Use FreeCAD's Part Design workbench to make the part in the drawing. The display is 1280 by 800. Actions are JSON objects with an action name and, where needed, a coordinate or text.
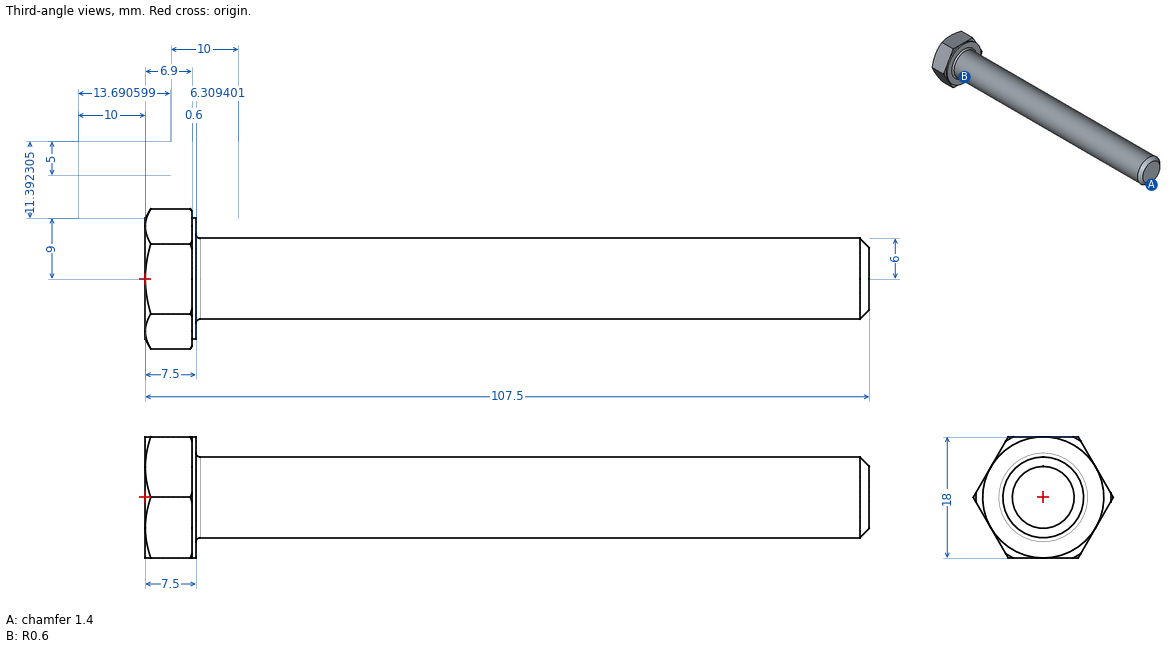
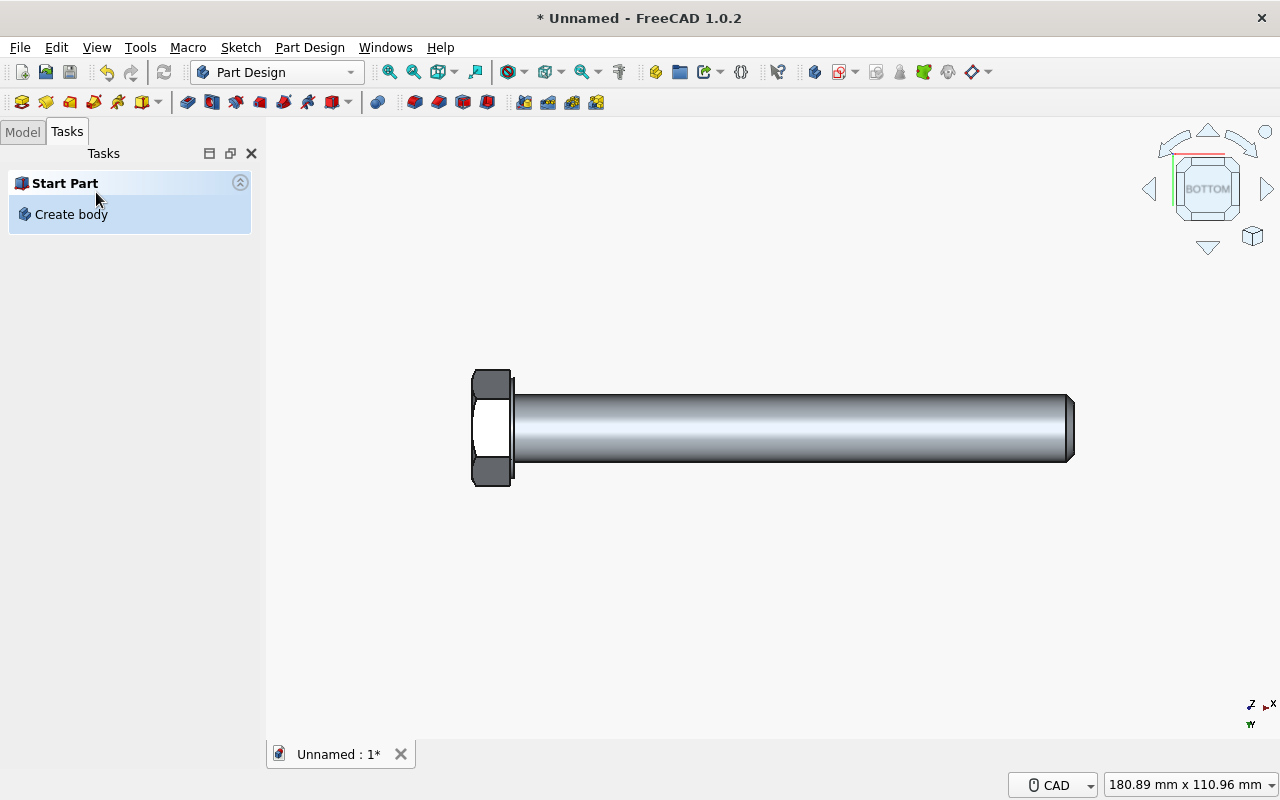
{"action": "key", "text": "4"}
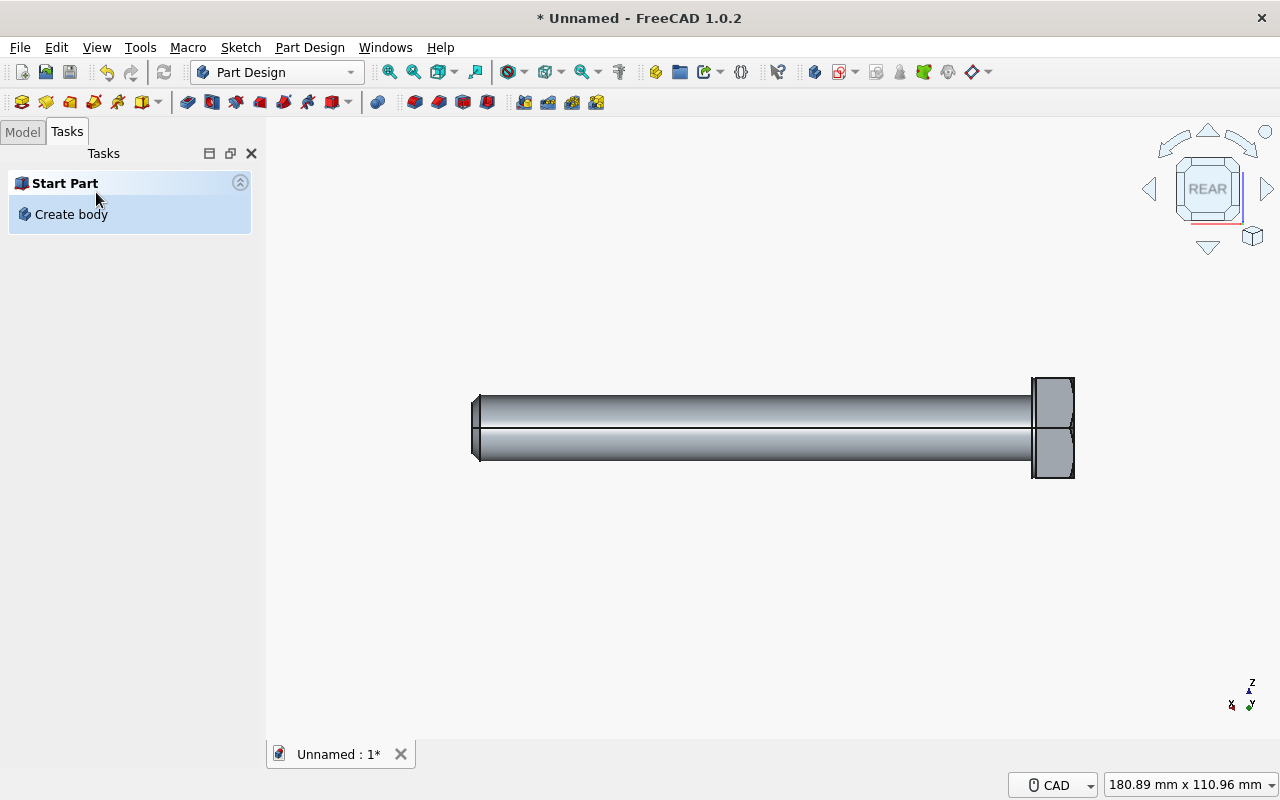
{"action": "key", "text": "6"}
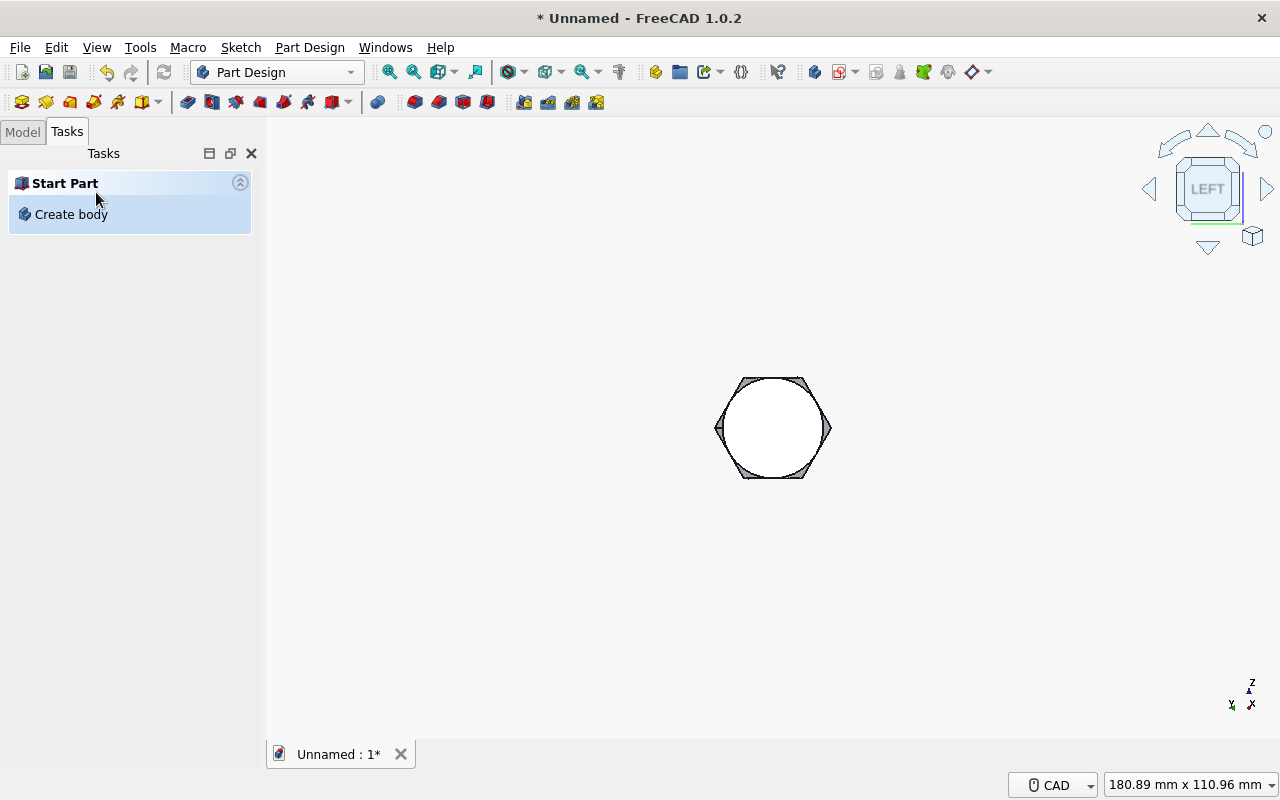
{"action": "key", "text": "v f"}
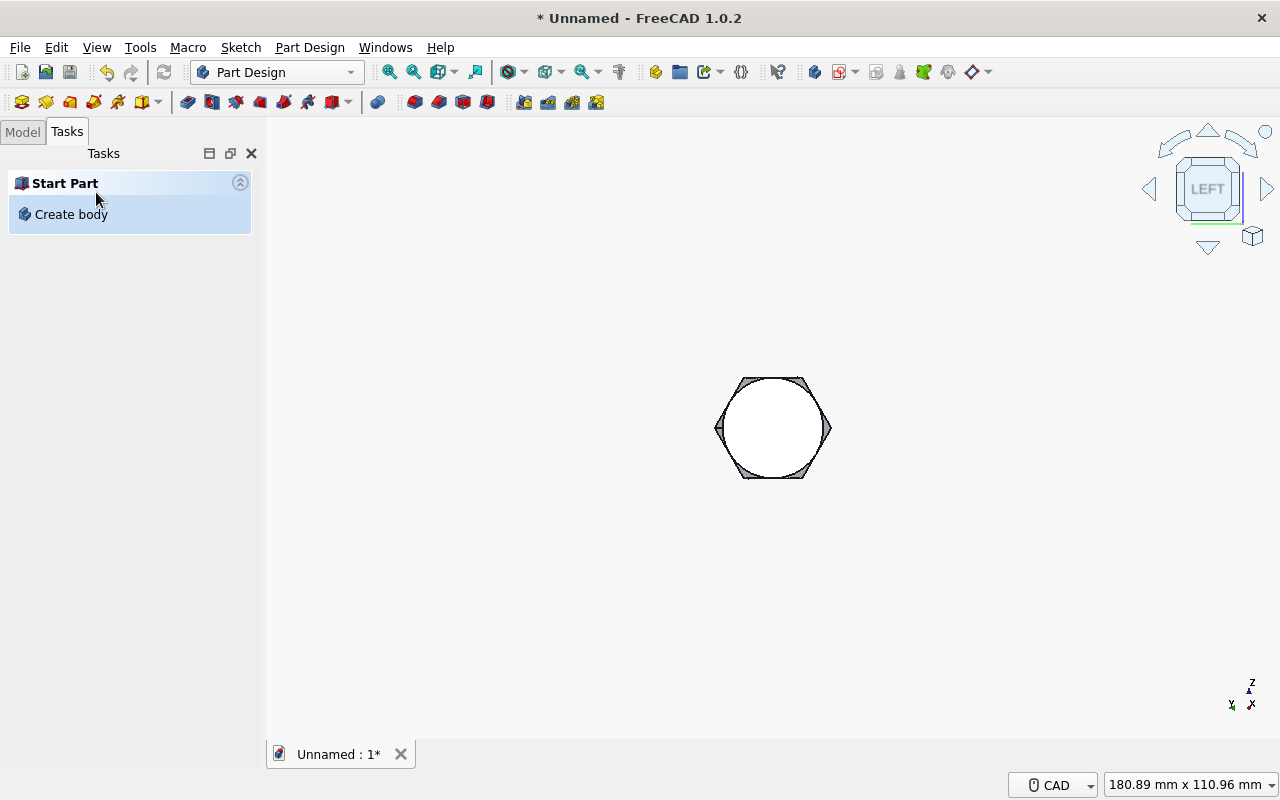
{"action": "key", "text": "v 3"}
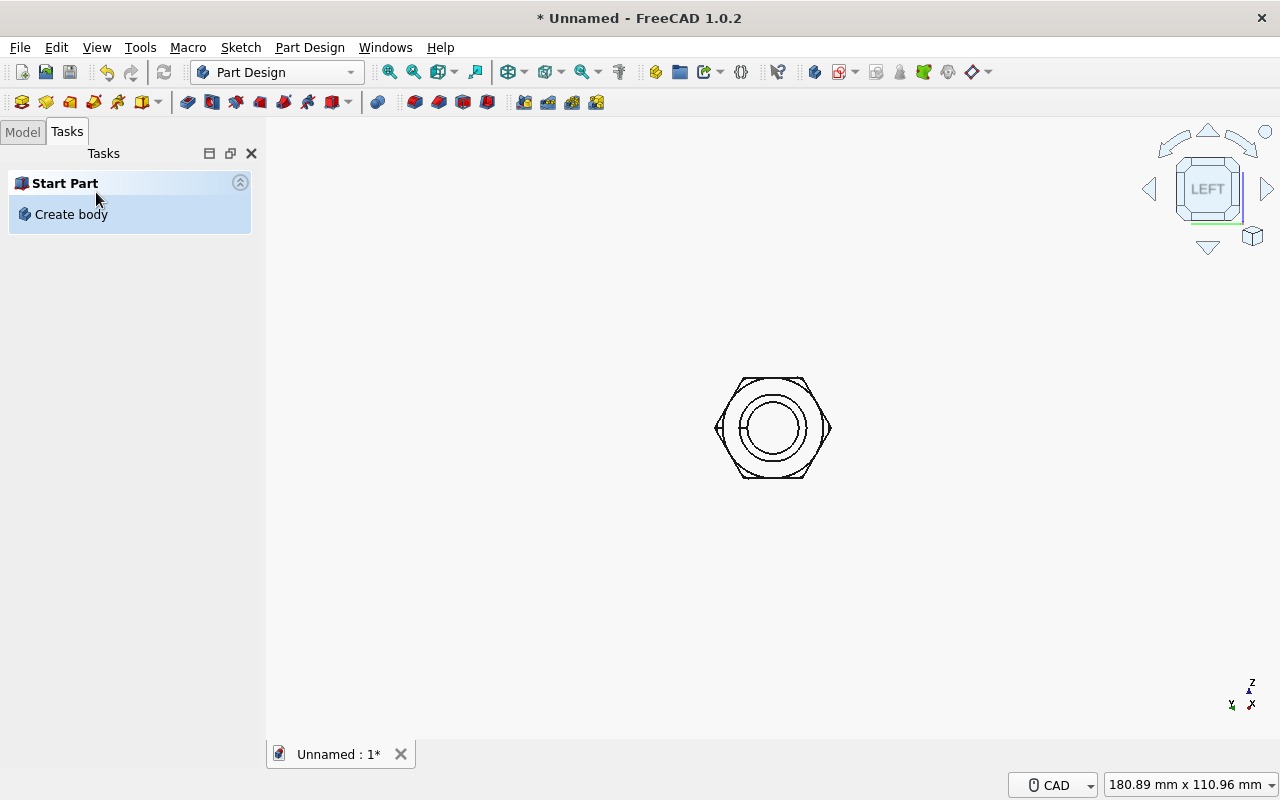
{"action": "key", "text": "0"}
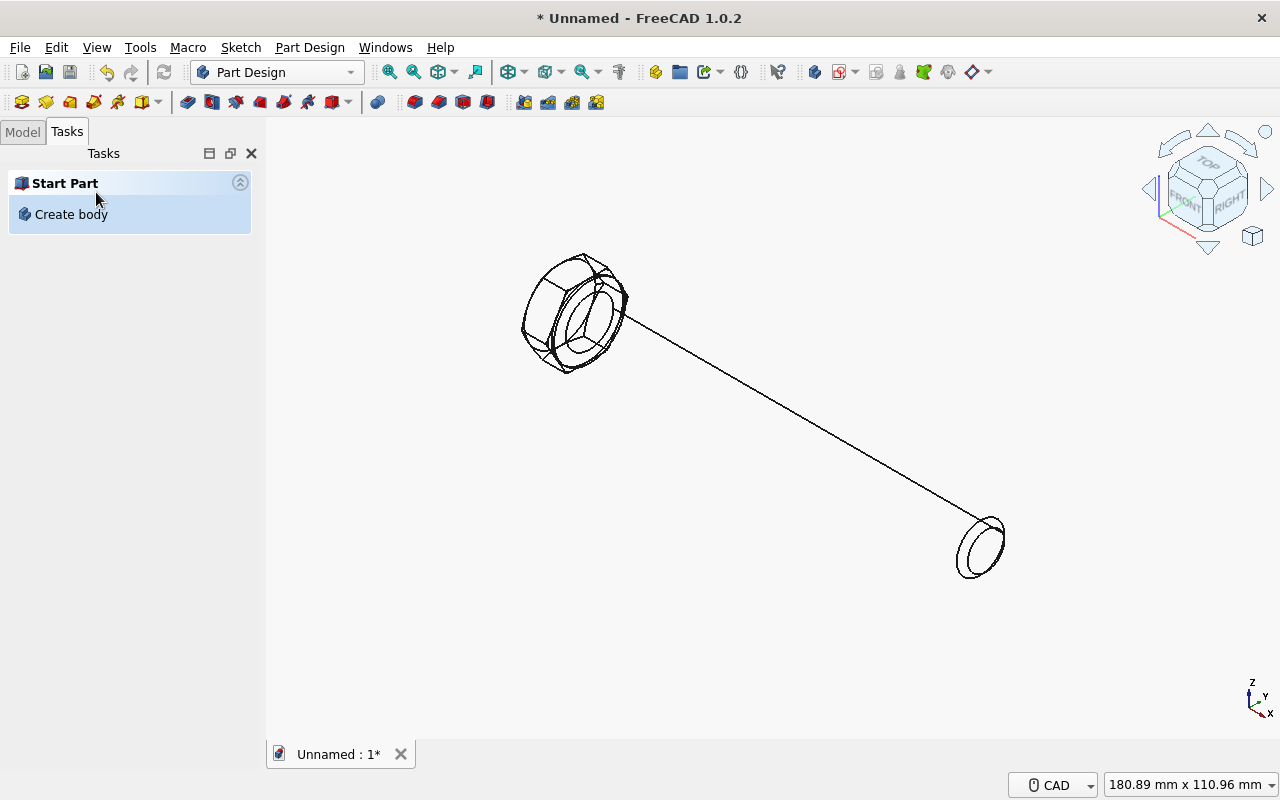
{"action": "left_click", "coordinate": [566, 335]}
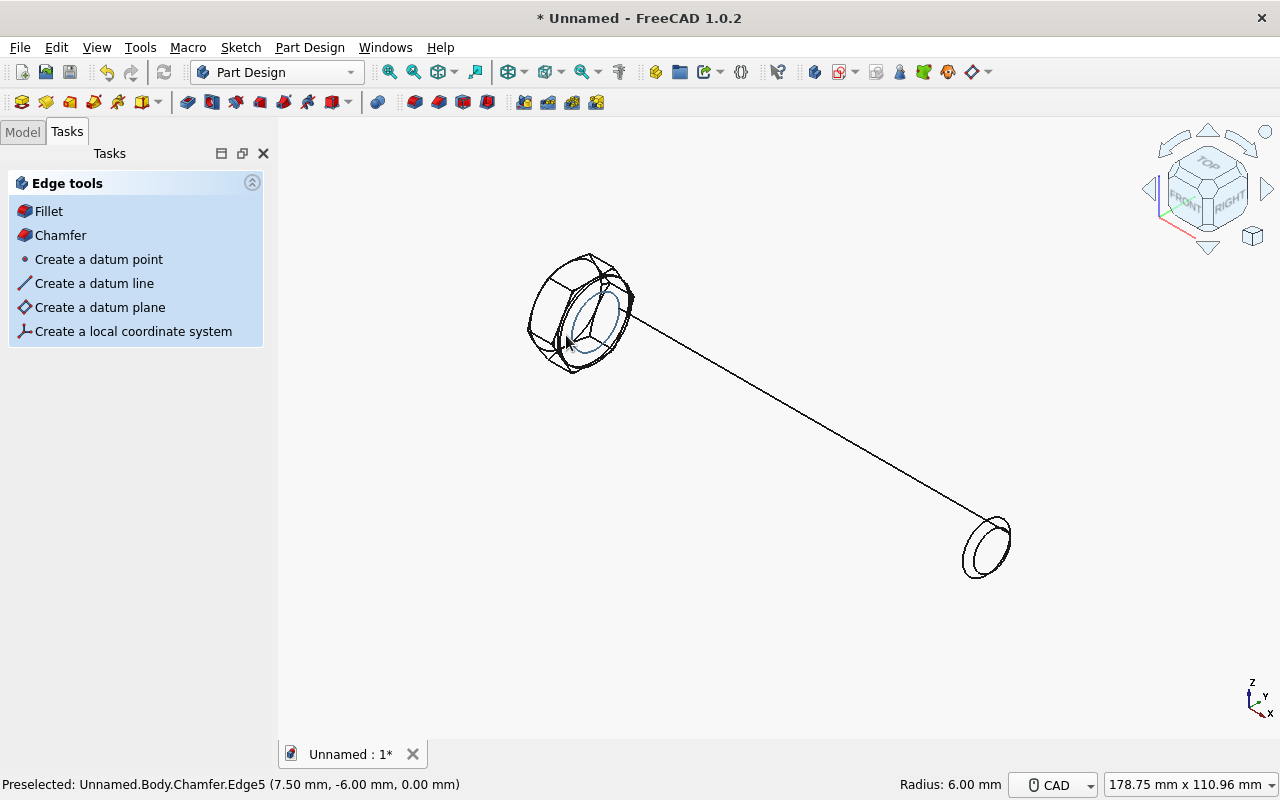
{"action": "key", "text": "v 1"}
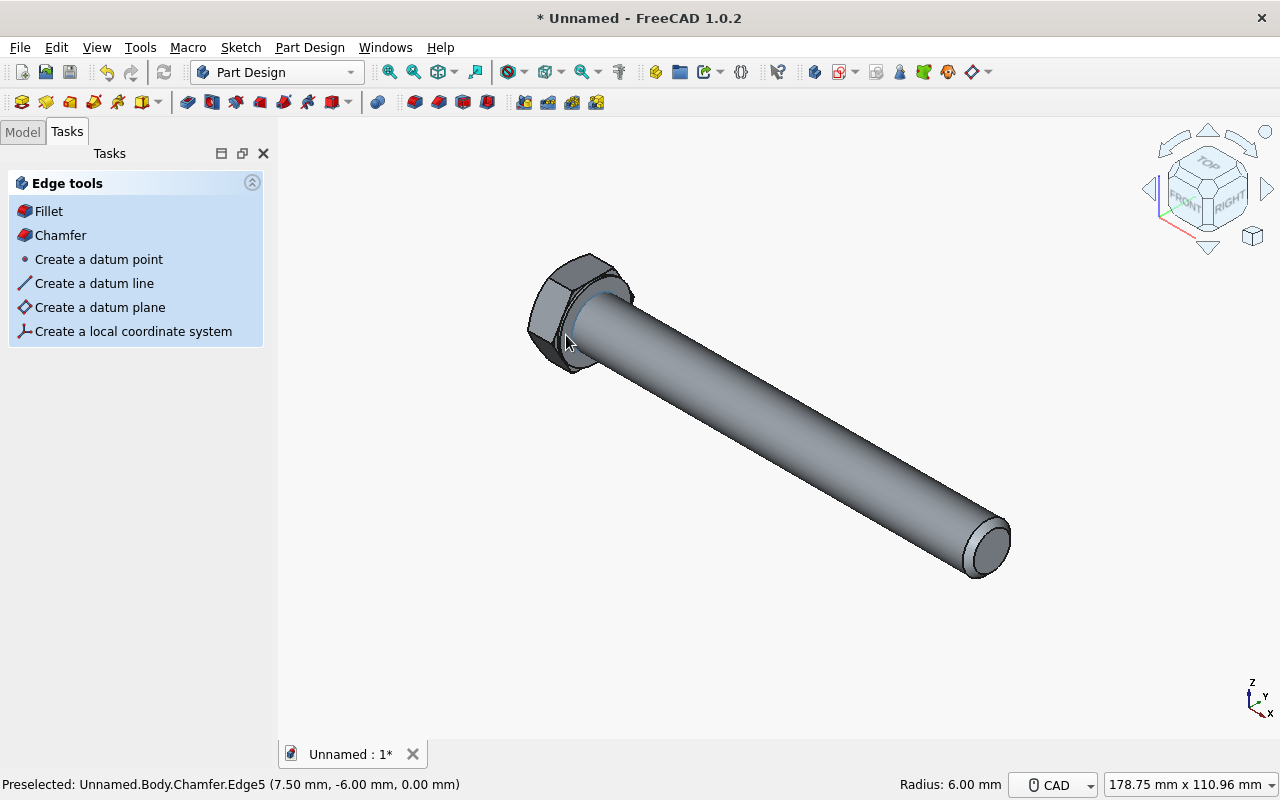
{"action": "left_click", "coordinate": [416, 102]}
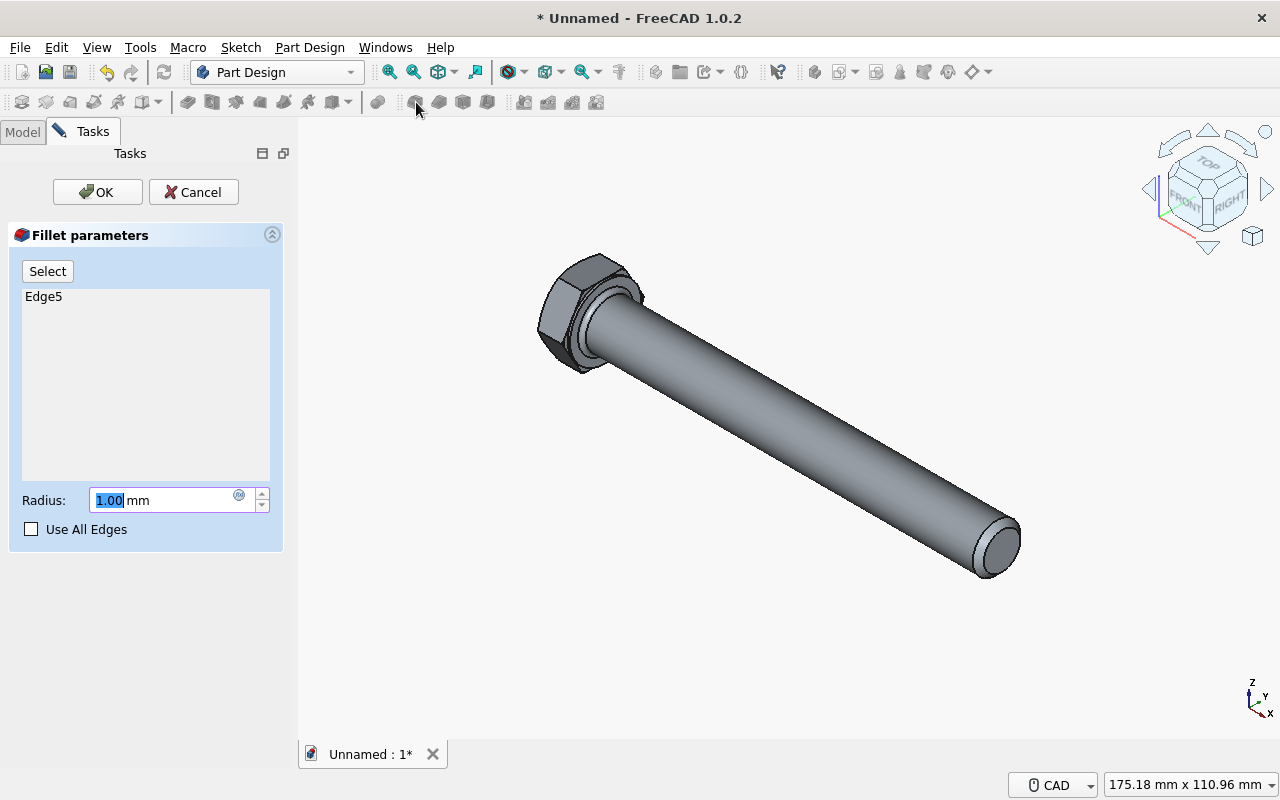
{"action": "type", "text": "0.6"}
{"action": "key", "text": "Tab"}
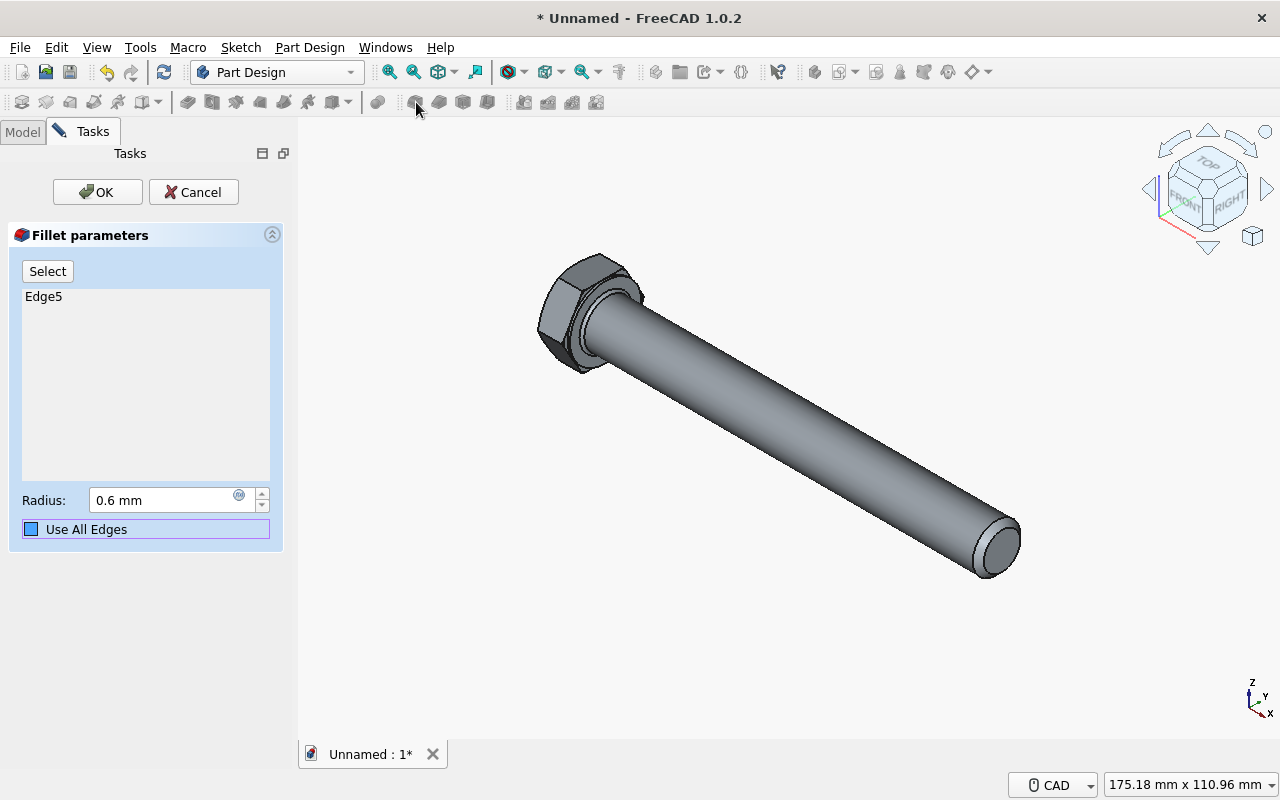
{"action": "left_click", "coordinate": [98, 192]}